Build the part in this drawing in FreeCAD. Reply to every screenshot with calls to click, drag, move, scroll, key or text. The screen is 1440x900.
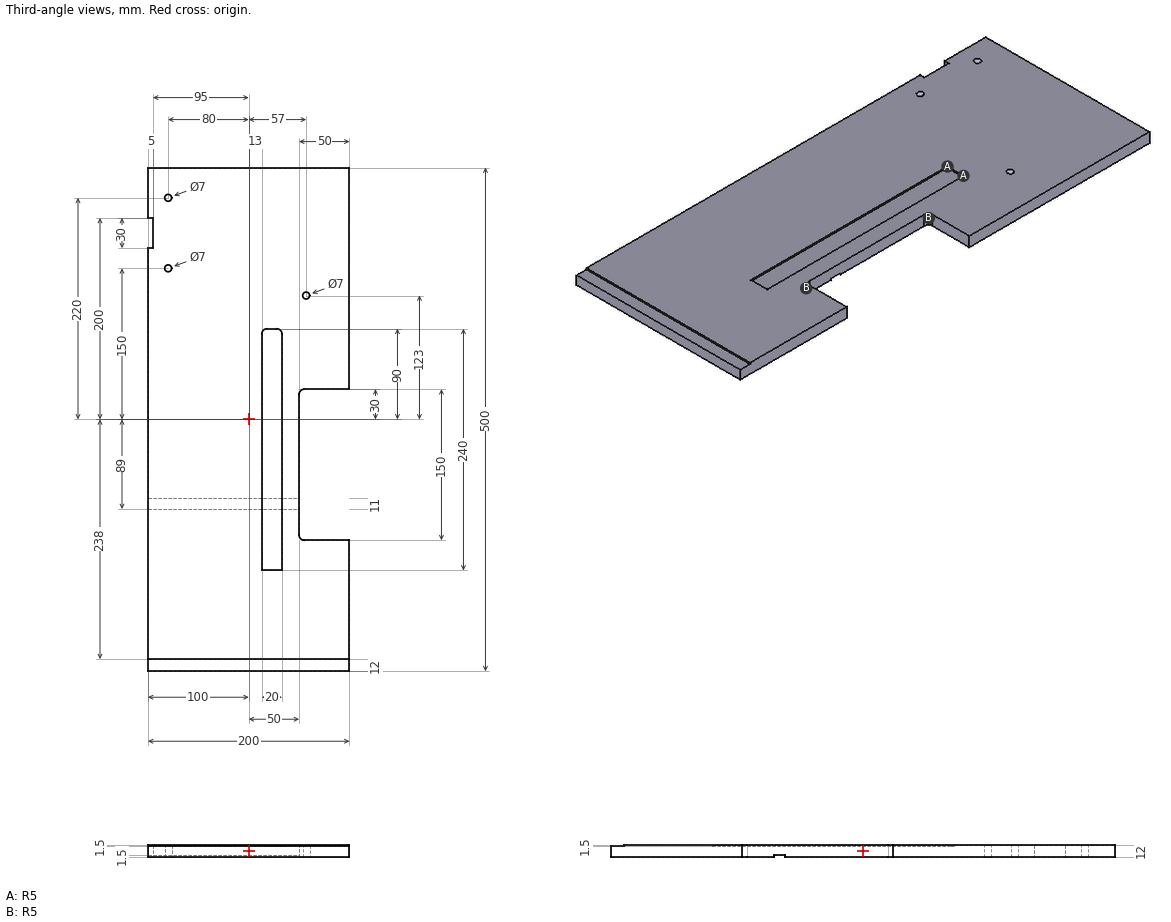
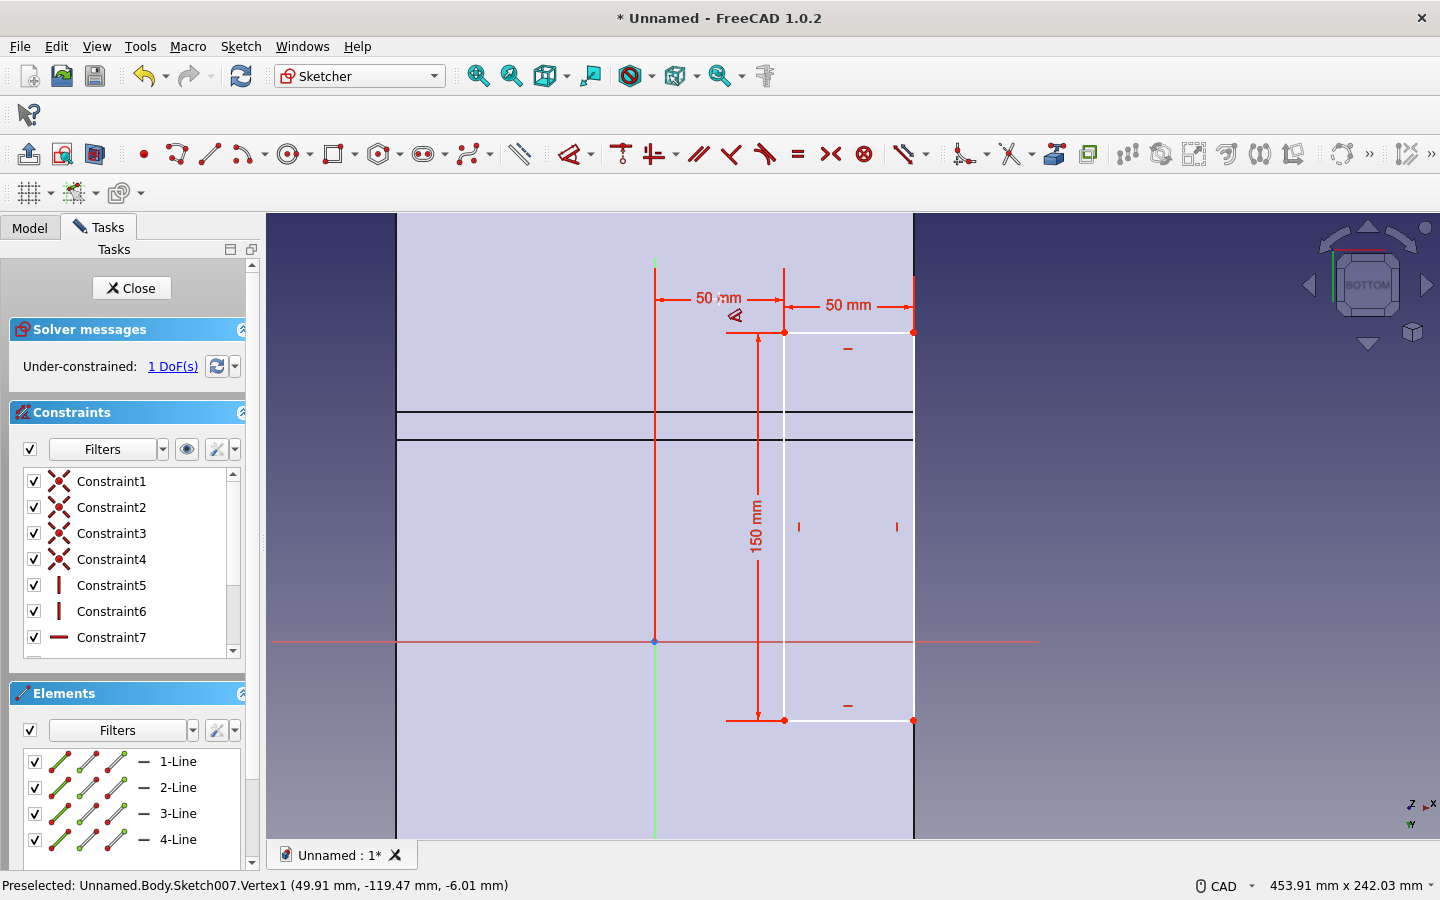
click(784, 721)
click(621, 681)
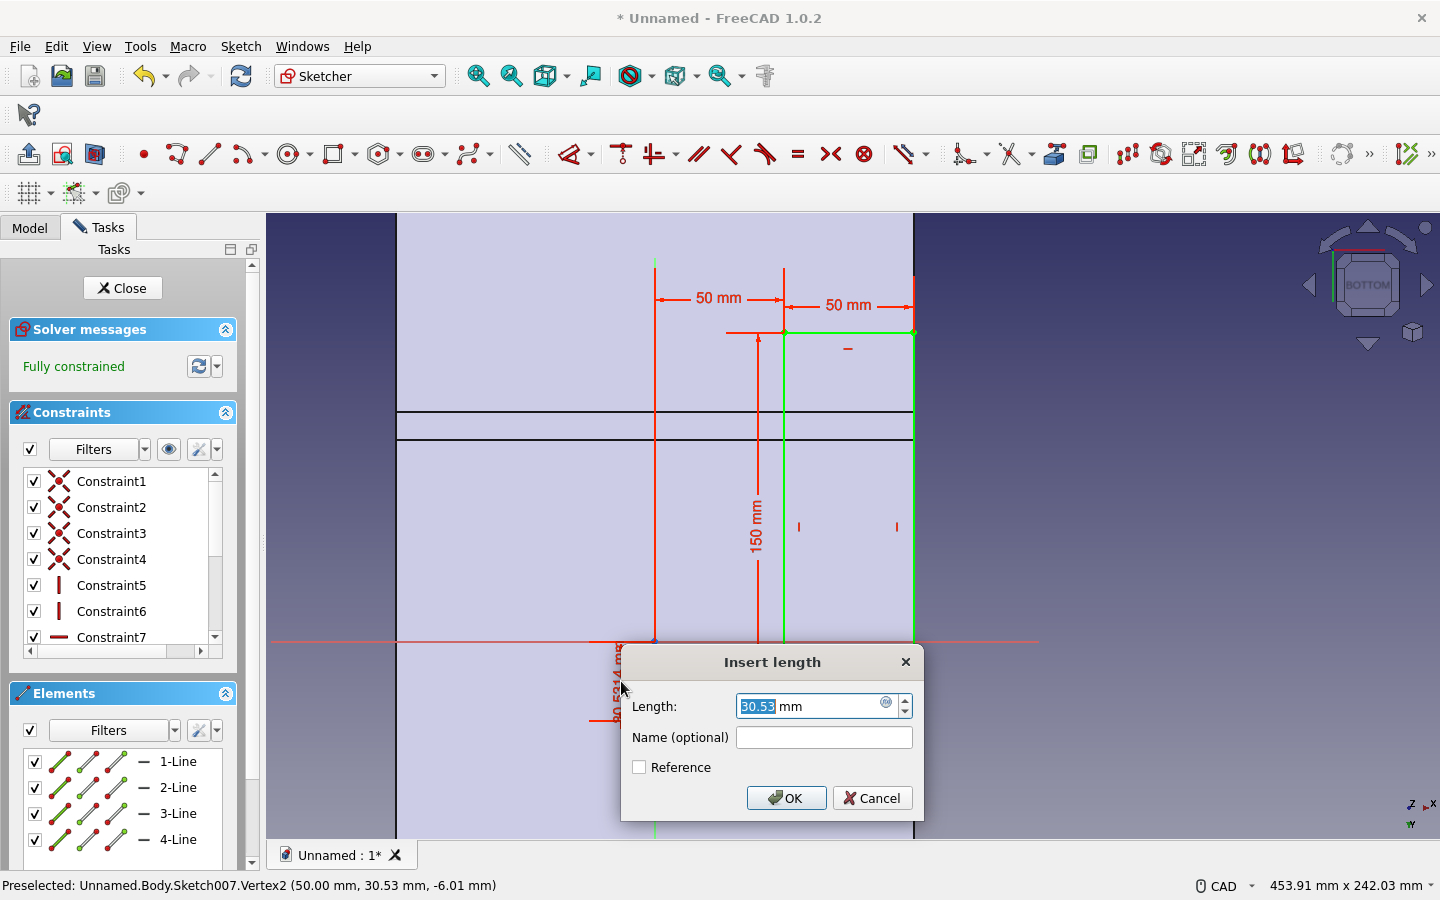
text(30)
key(Return)
key(Escape)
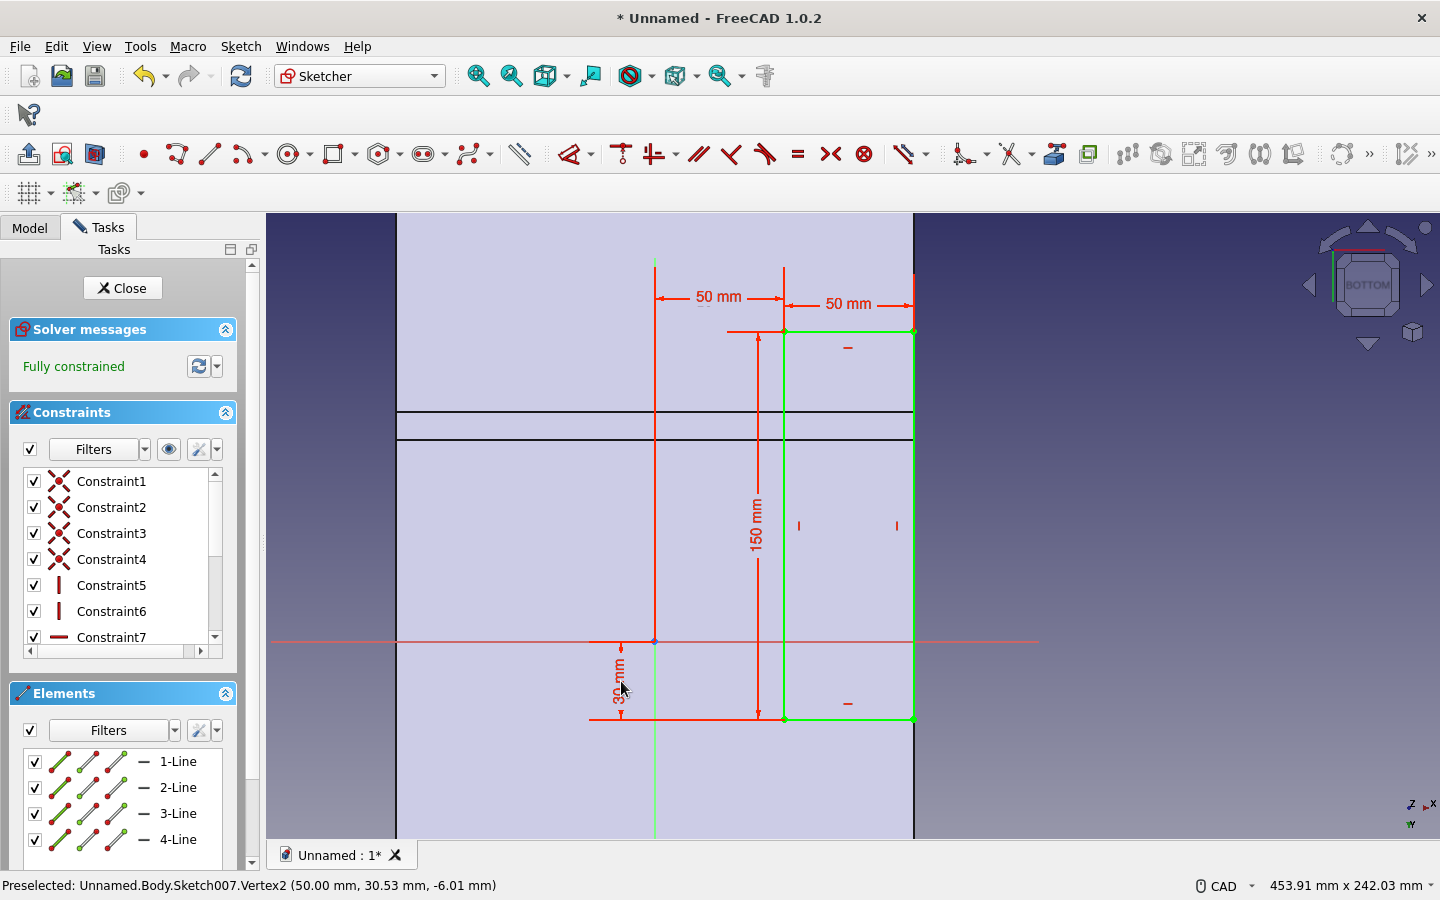
click(123, 288)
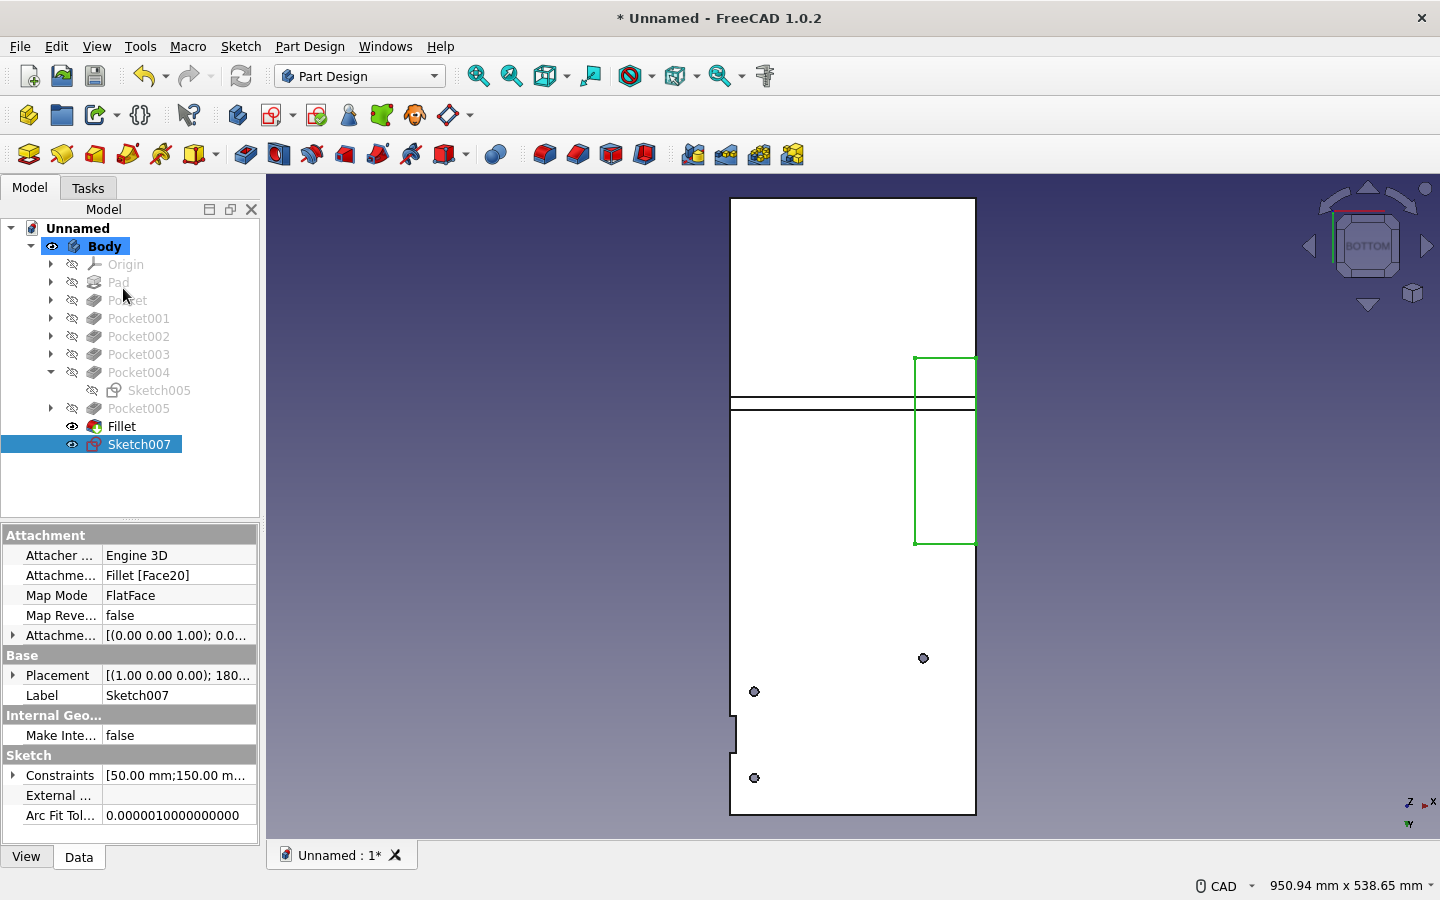
click(246, 154)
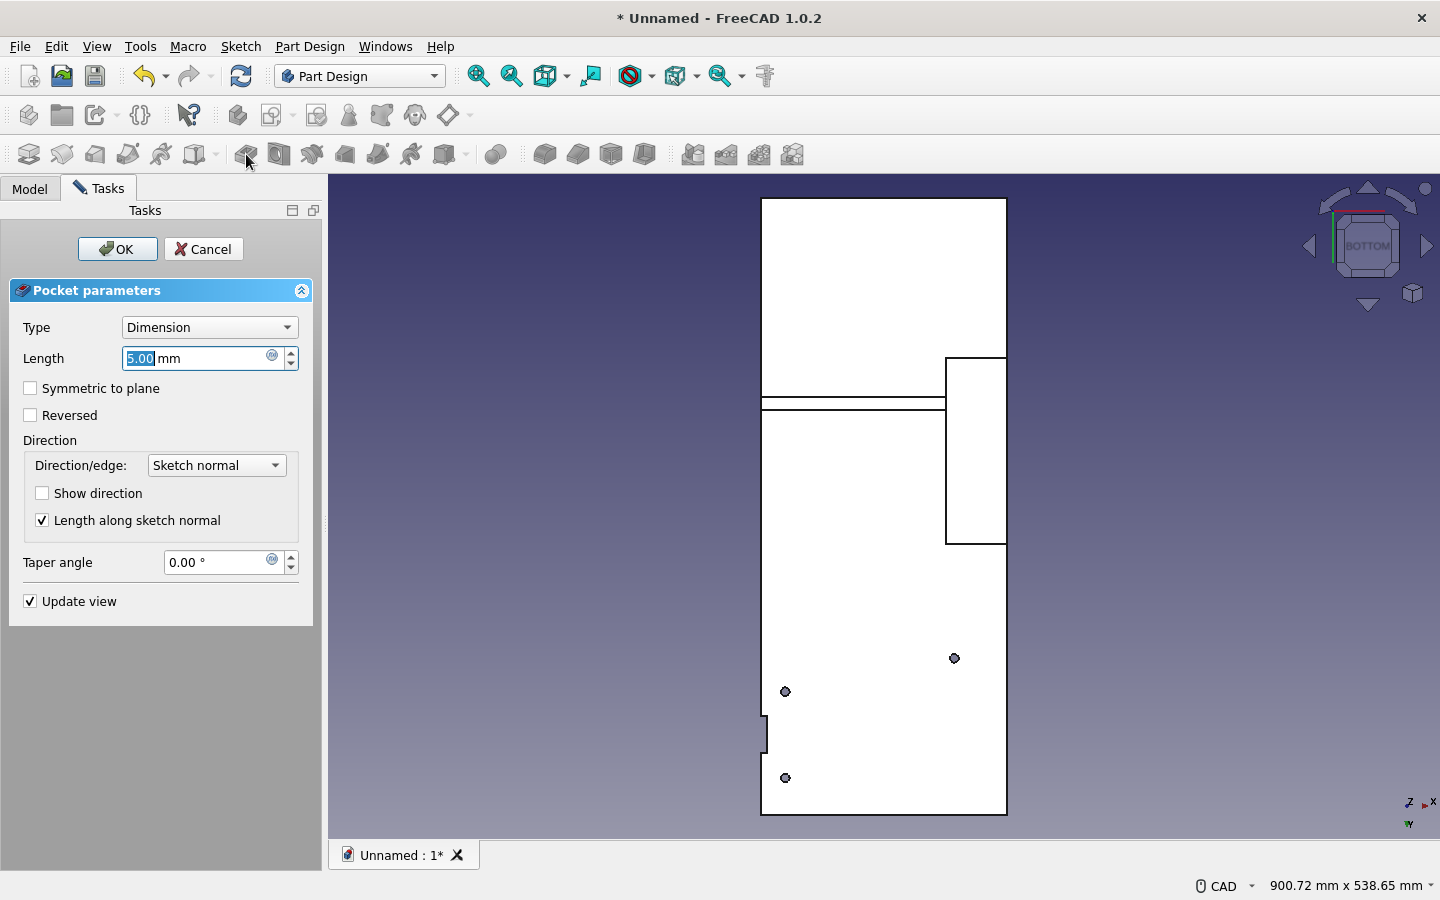
click(210, 328)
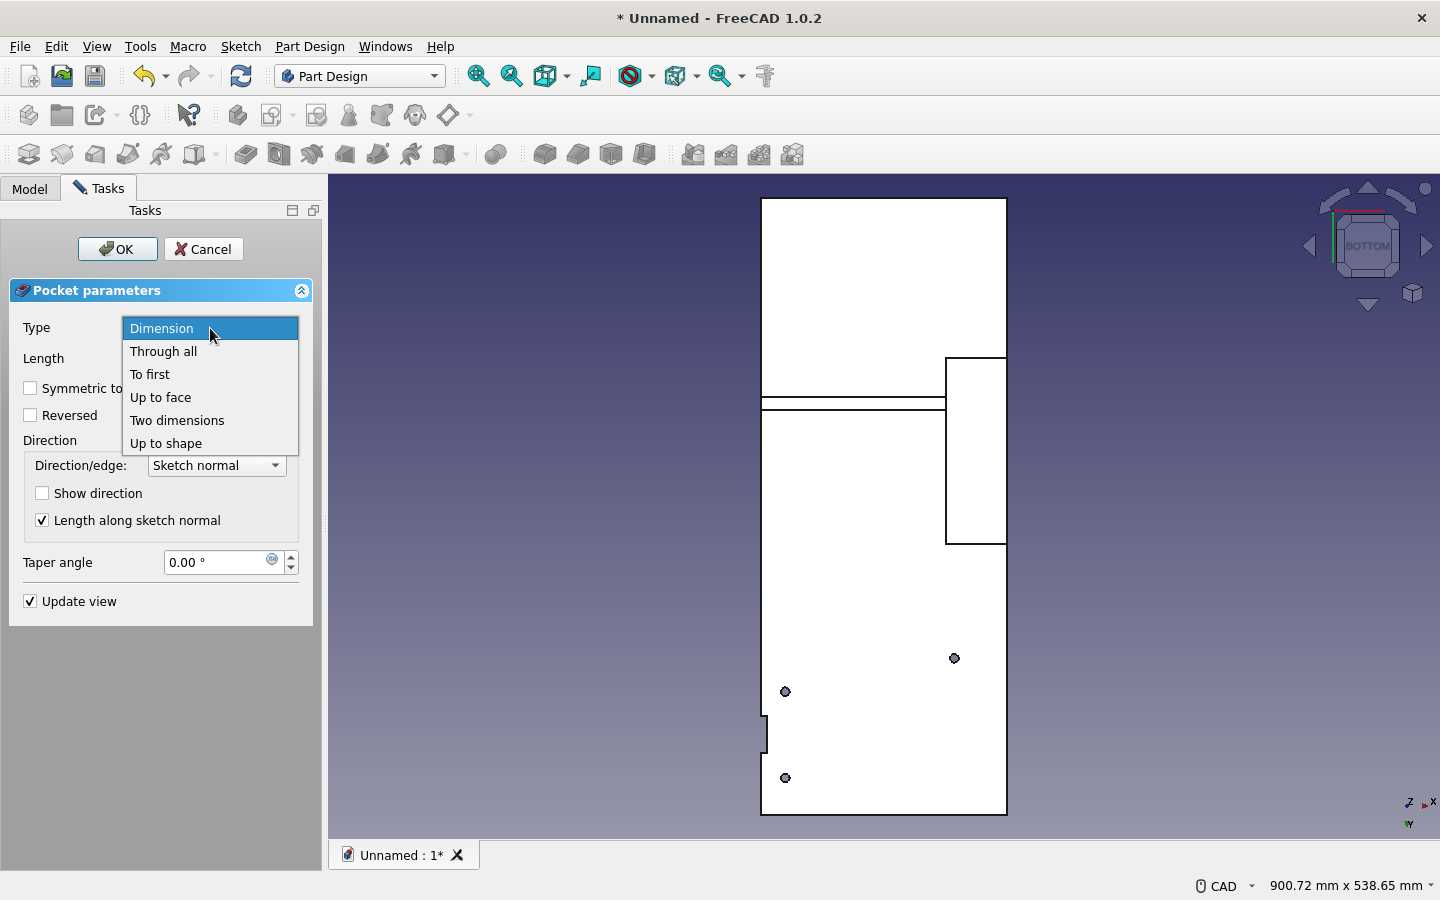
click(208, 374)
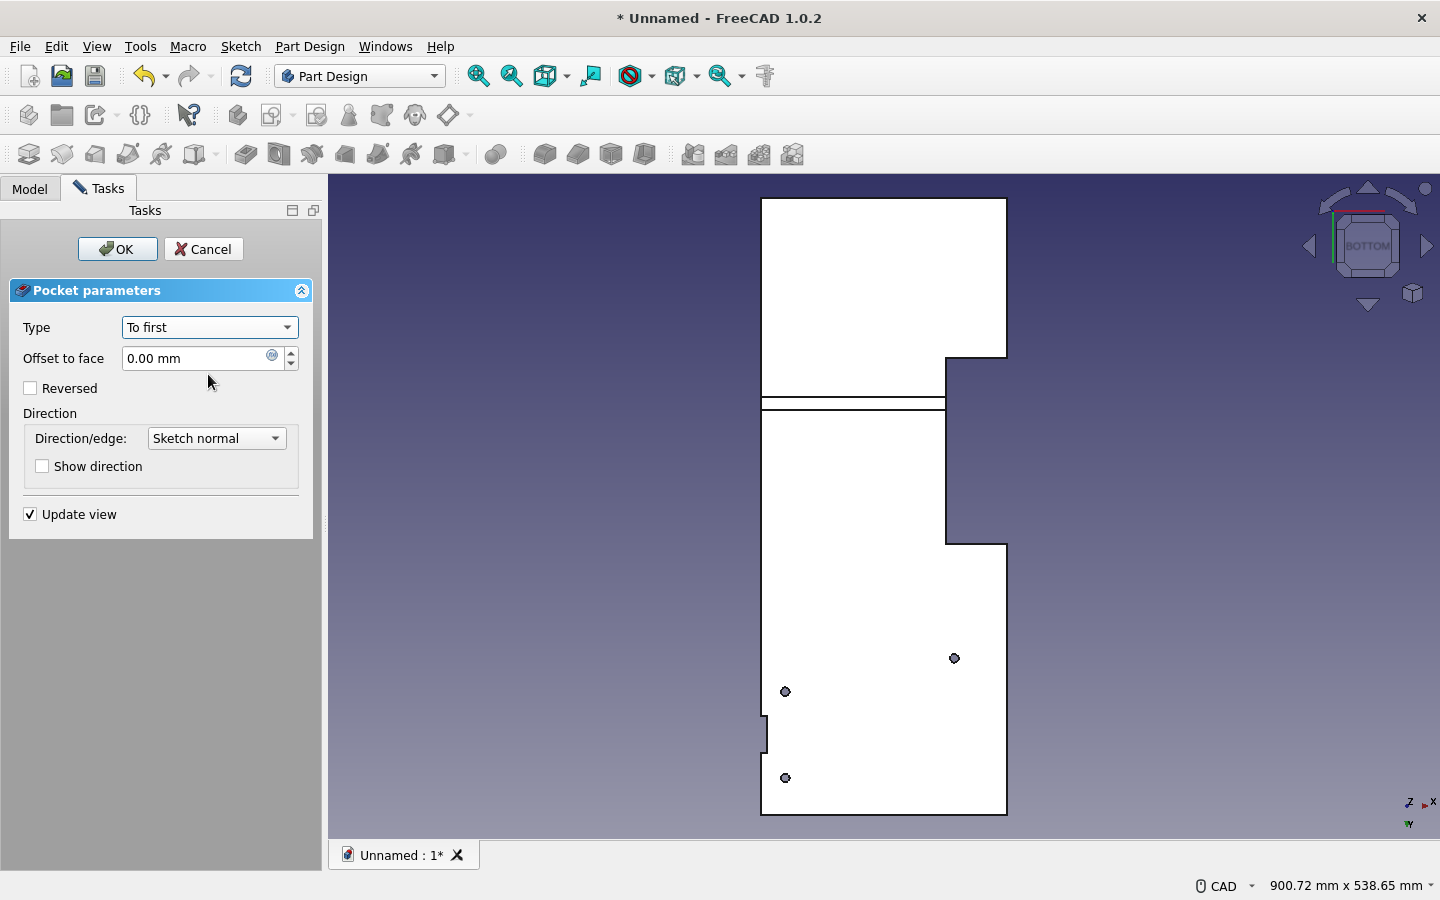
click(118, 249)